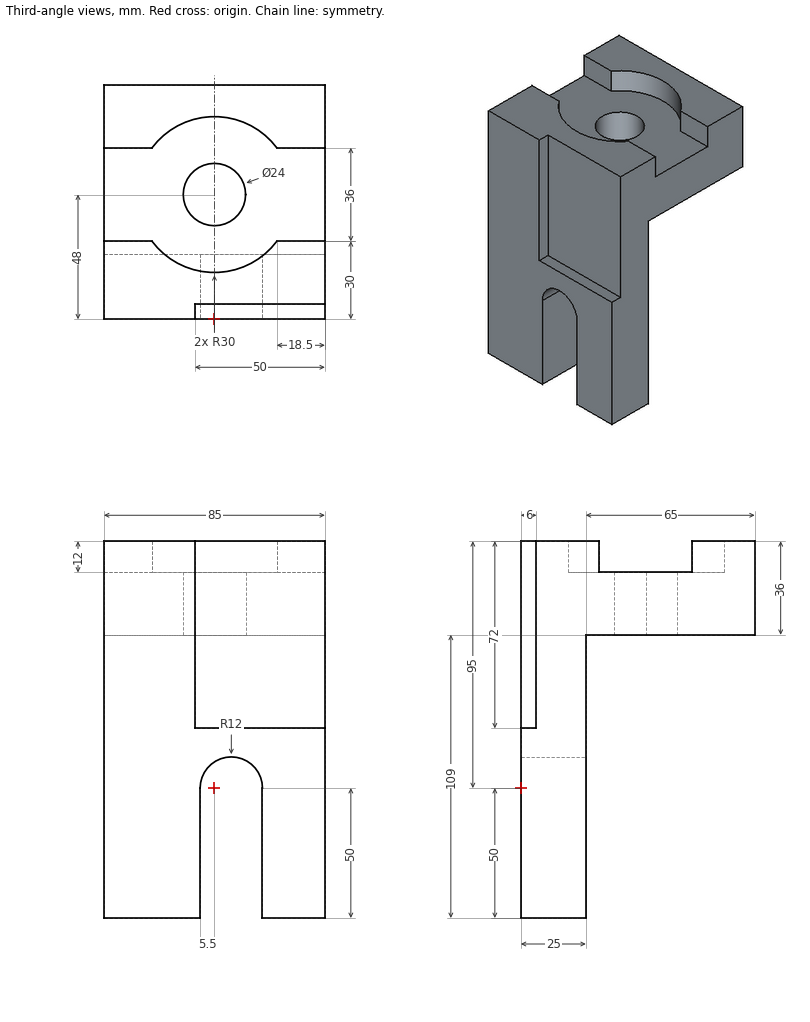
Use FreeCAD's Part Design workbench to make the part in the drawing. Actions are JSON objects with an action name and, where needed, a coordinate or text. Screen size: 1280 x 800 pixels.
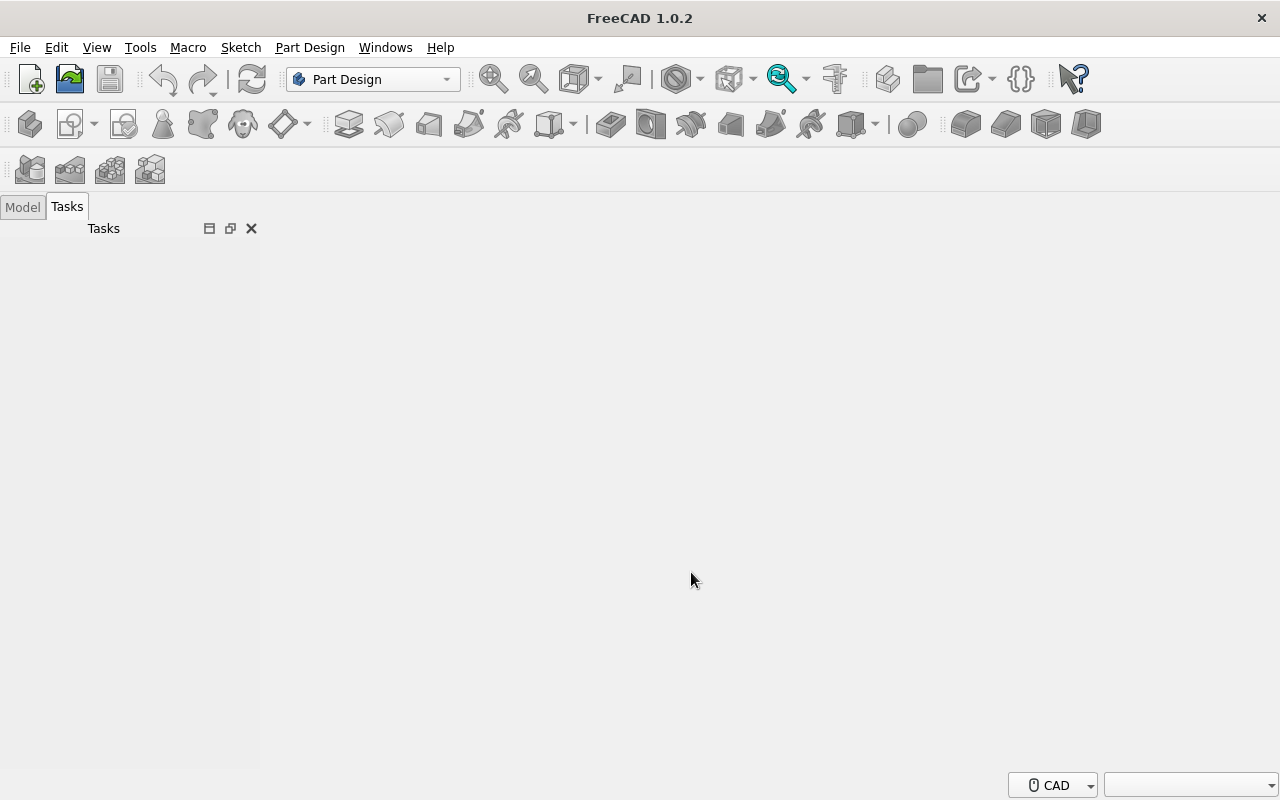
{"action": "left_click", "coordinate": [30, 80]}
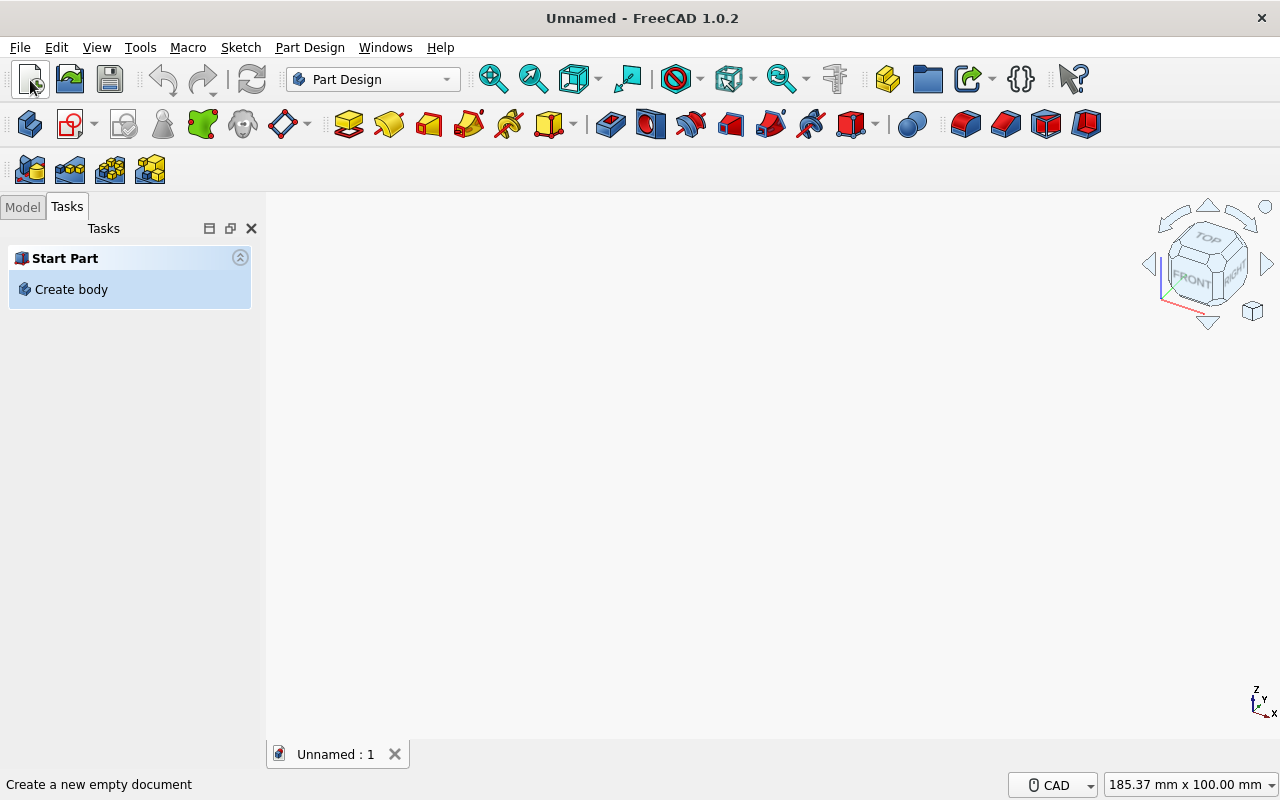
{"action": "left_click", "coordinate": [70, 124]}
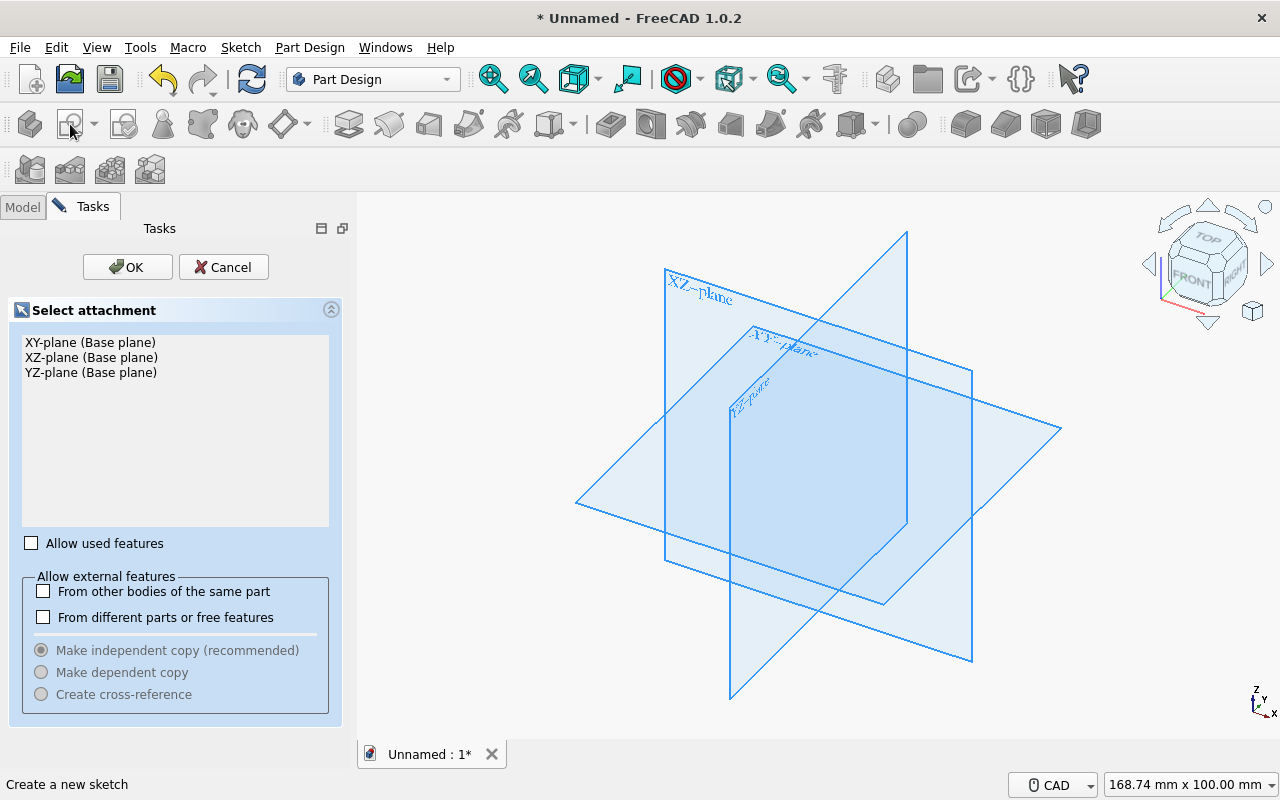
{"action": "left_click", "coordinate": [82, 372]}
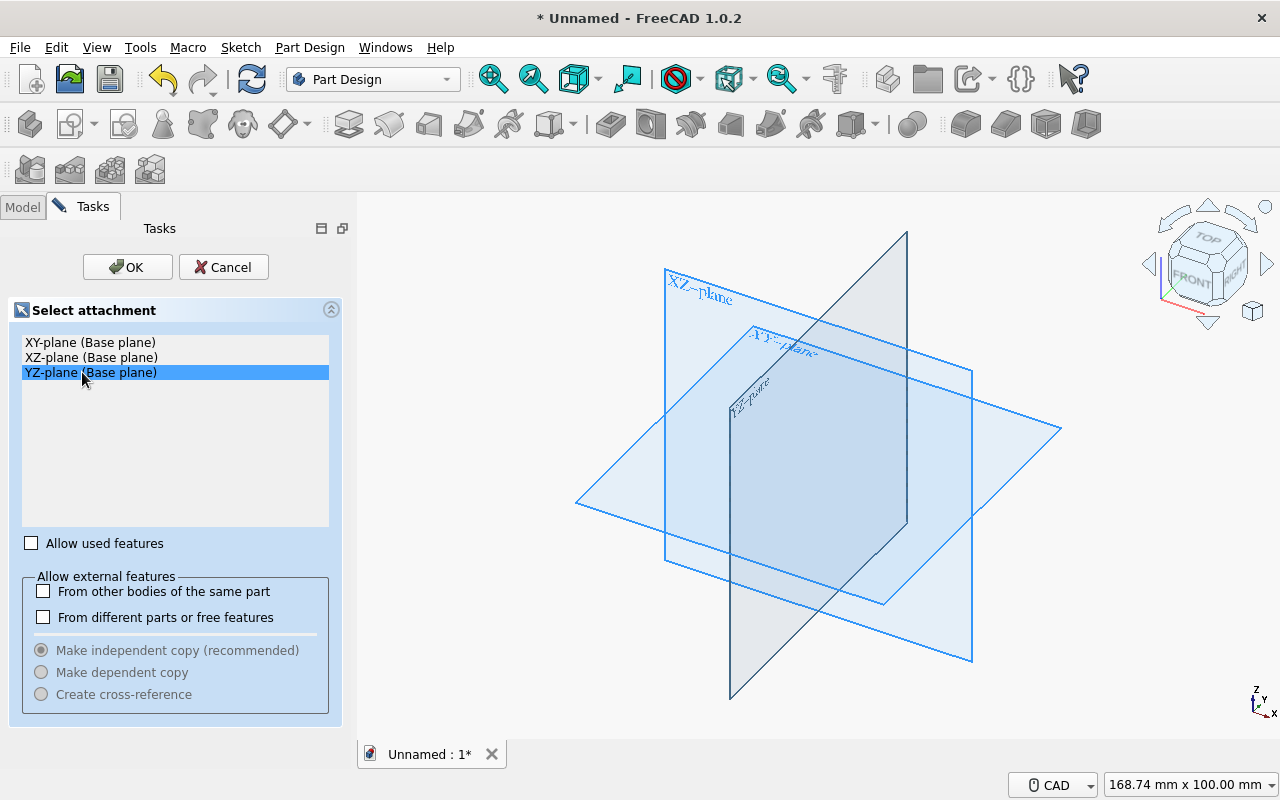
{"action": "left_click", "coordinate": [128, 267]}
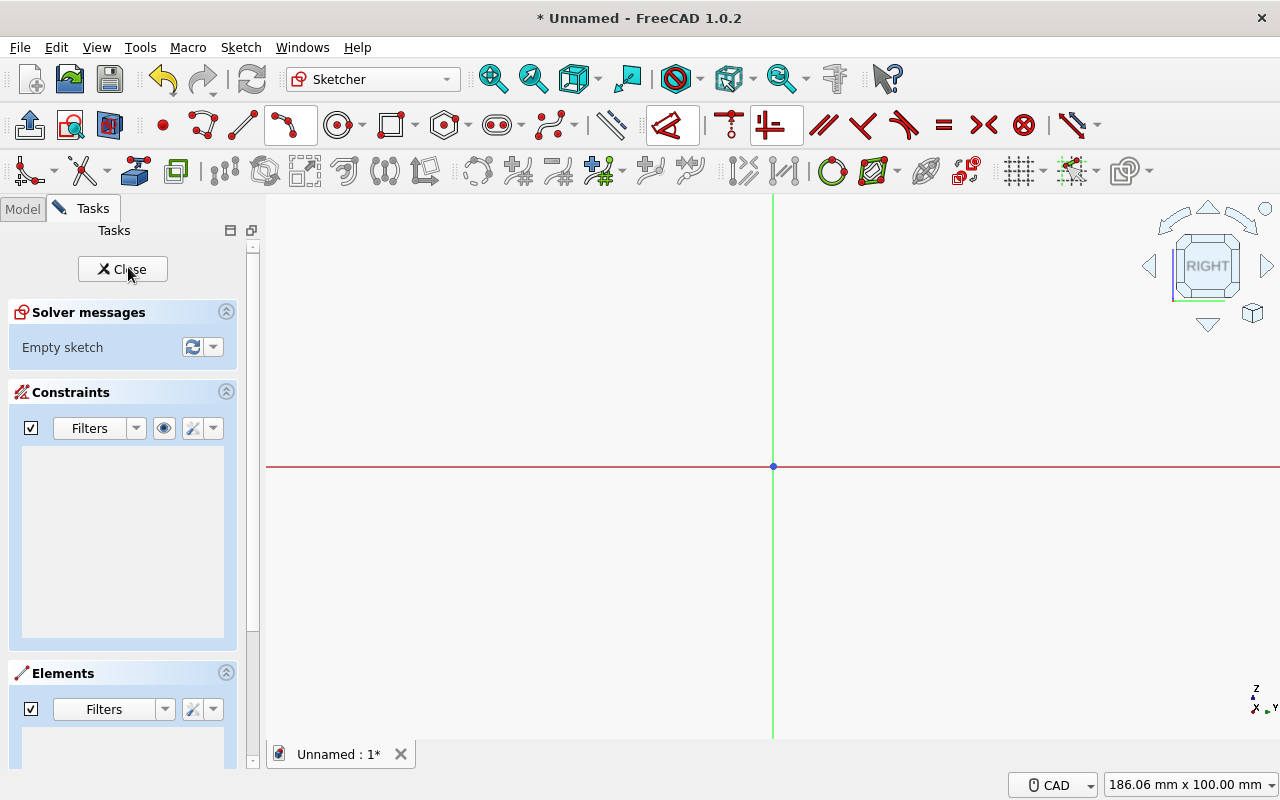
{"action": "scroll", "coordinate": [448, 567], "scroll_direction": "down", "scroll_amount": 4}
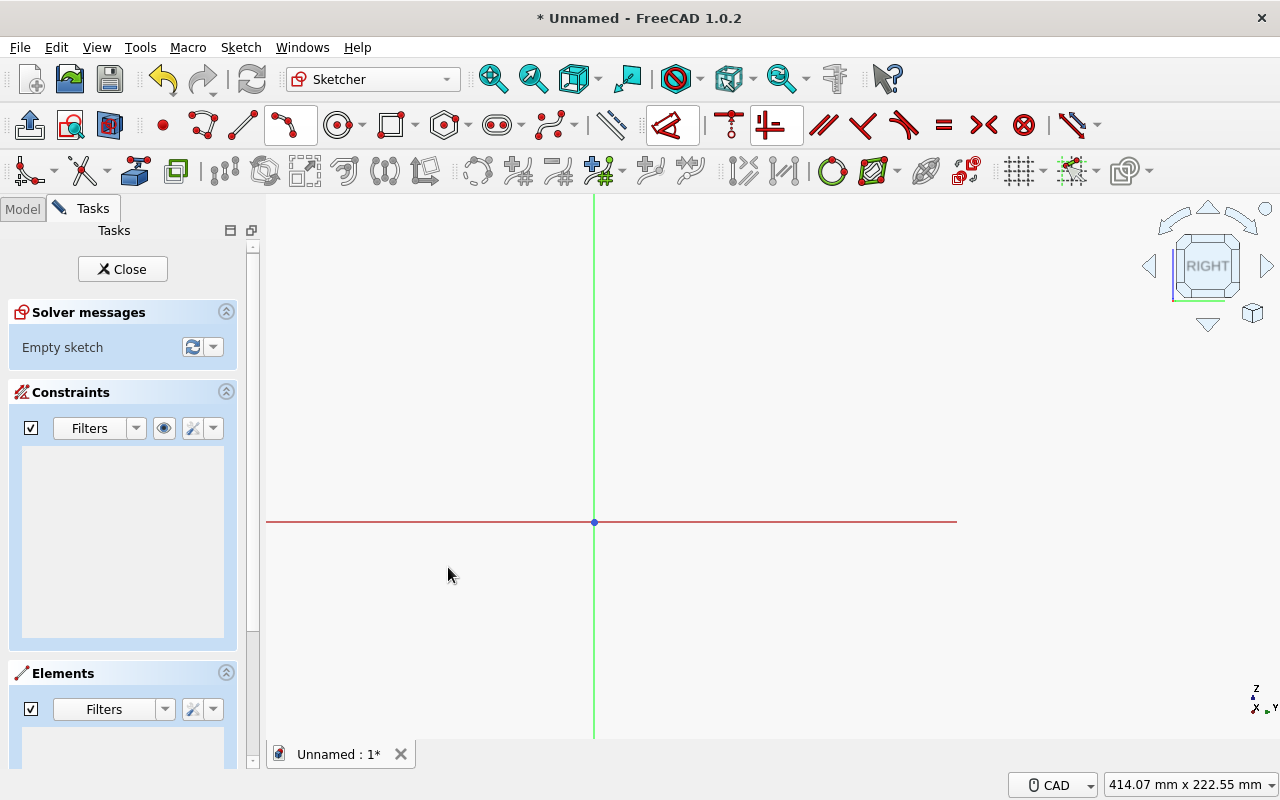
{"action": "left_click", "coordinate": [204, 126]}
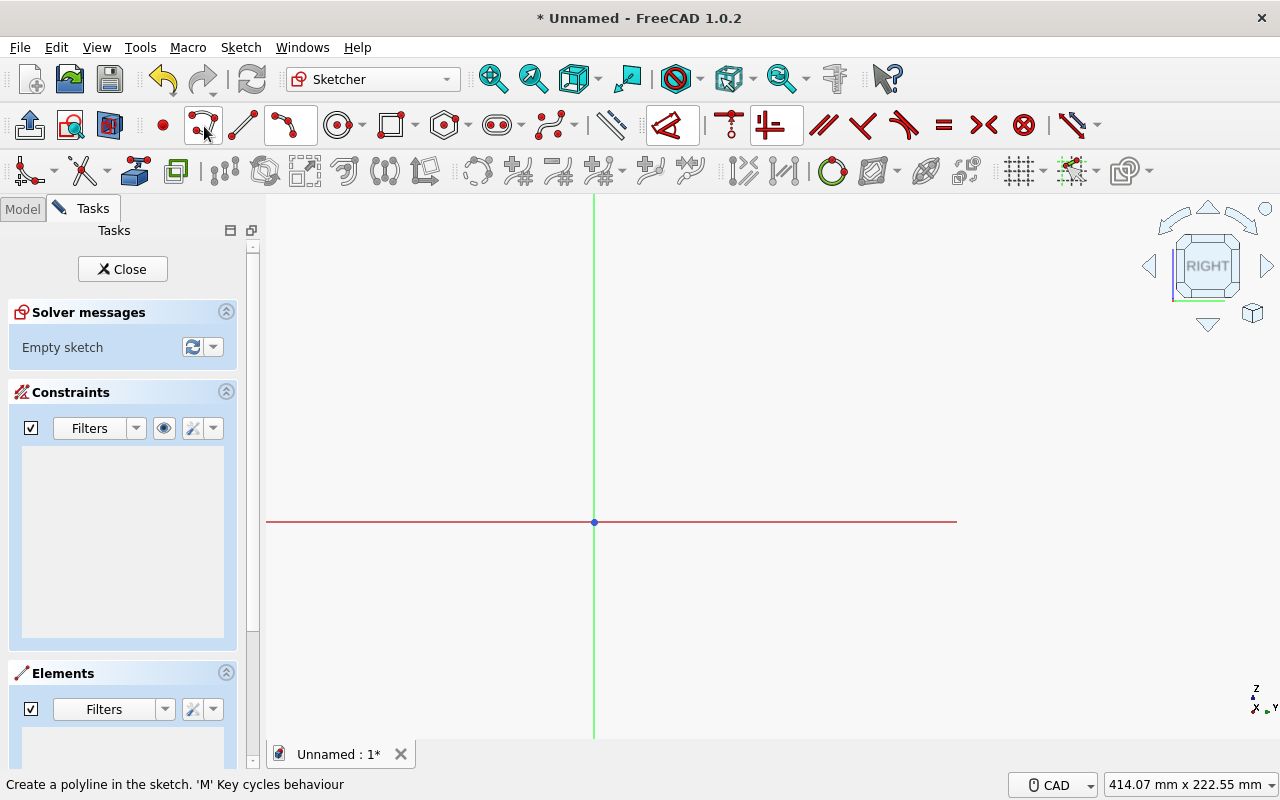
{"action": "left_click", "coordinate": [594, 645]}
{"action": "left_click", "coordinate": [655, 645]}
{"action": "left_click", "coordinate": [655, 378]}
{"action": "left_click", "coordinate": [815, 378]}
{"action": "left_click", "coordinate": [815, 290]}
{"action": "left_click", "coordinate": [603, 290]}
{"action": "left_click", "coordinate": [594, 646]}
{"action": "key", "text": "Escape"}
{"action": "key", "text": "Escape"}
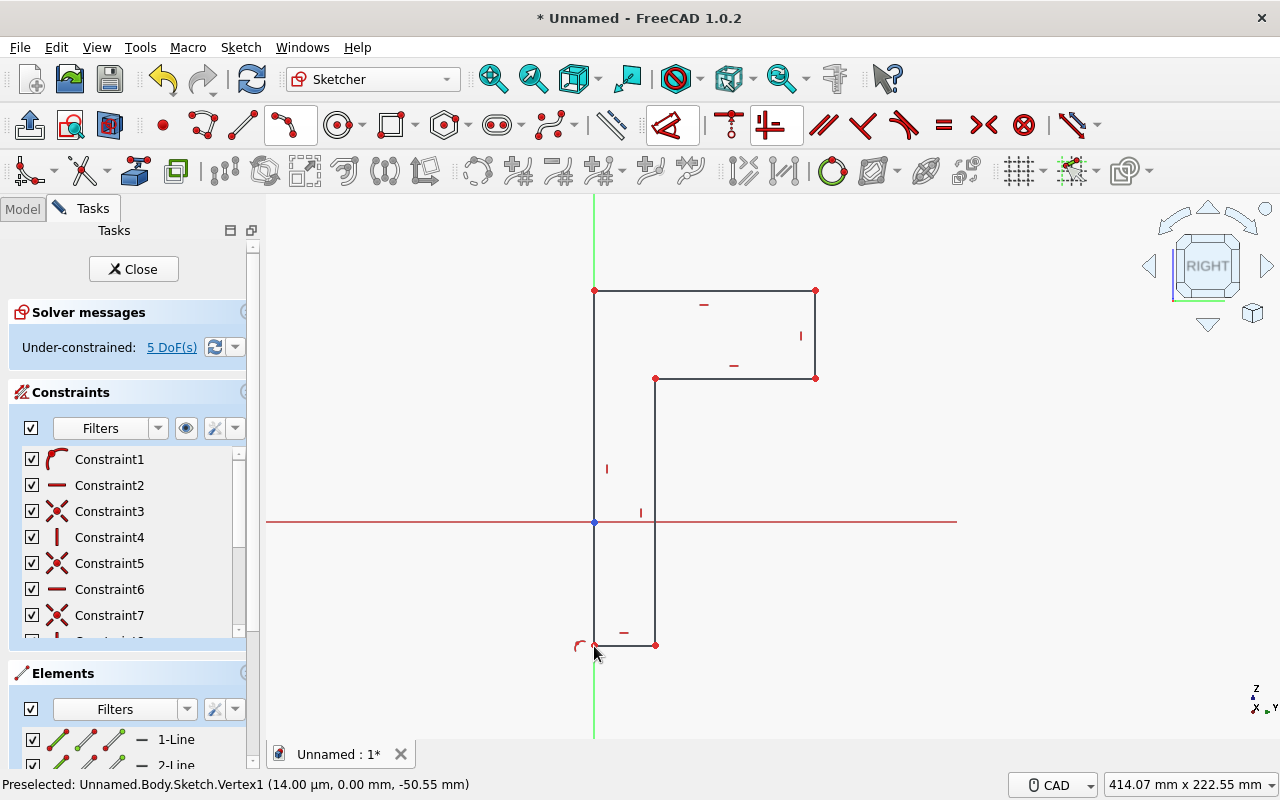
{"action": "left_click", "coordinate": [612, 646]}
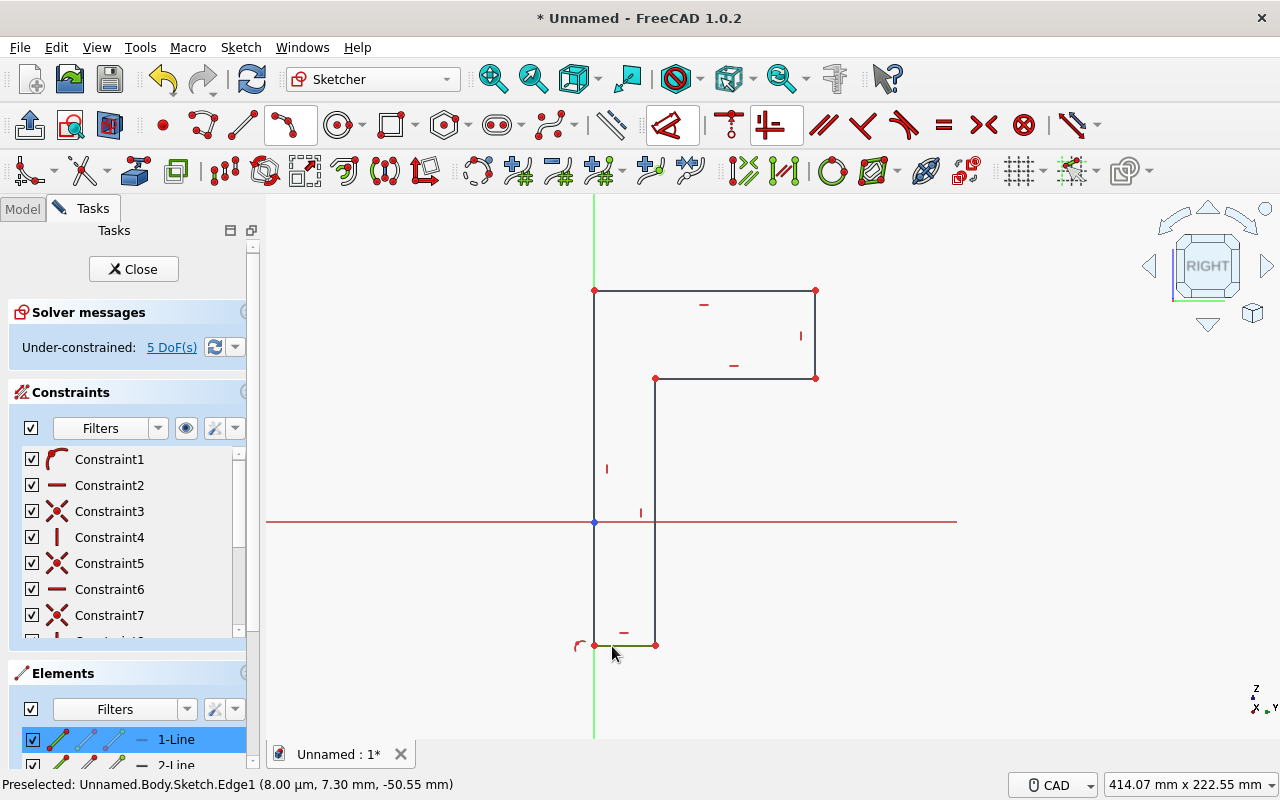
{"action": "left_click", "coordinate": [694, 126]}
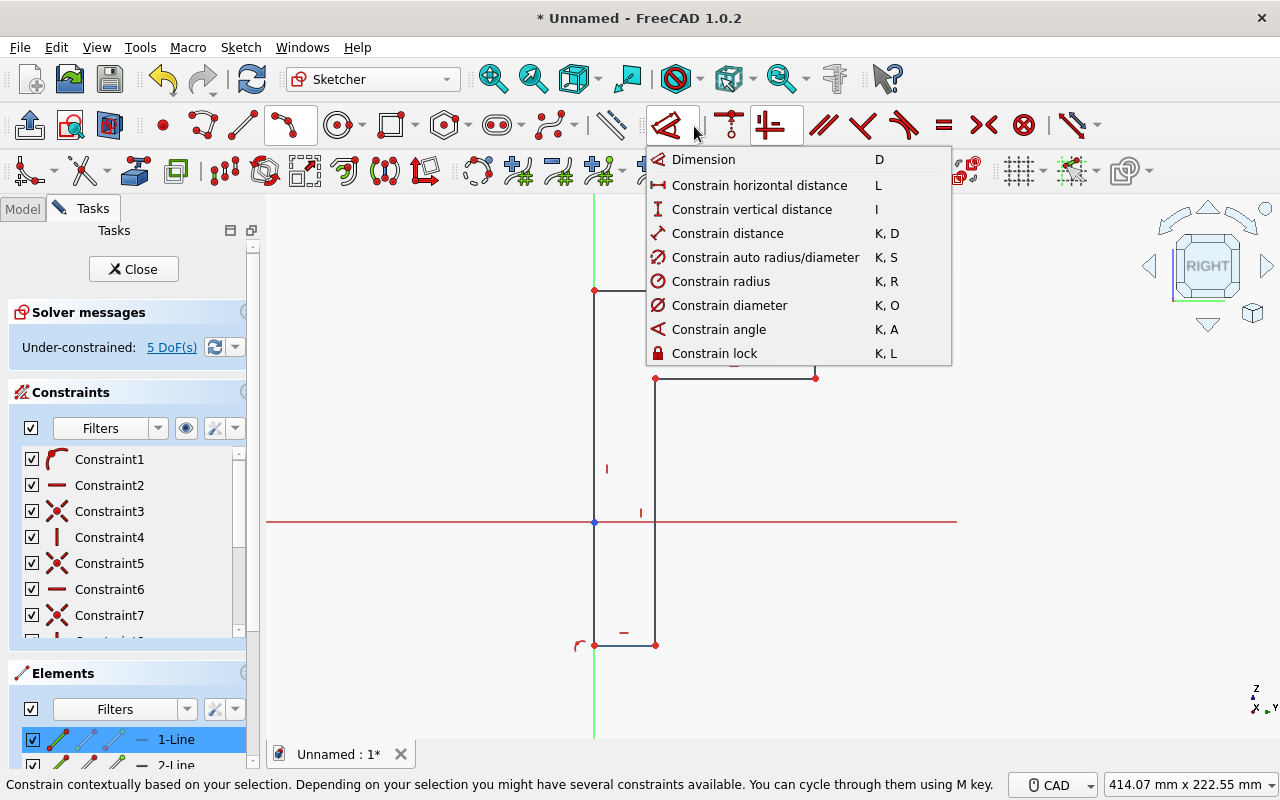
{"action": "left_click", "coordinate": [799, 185]}